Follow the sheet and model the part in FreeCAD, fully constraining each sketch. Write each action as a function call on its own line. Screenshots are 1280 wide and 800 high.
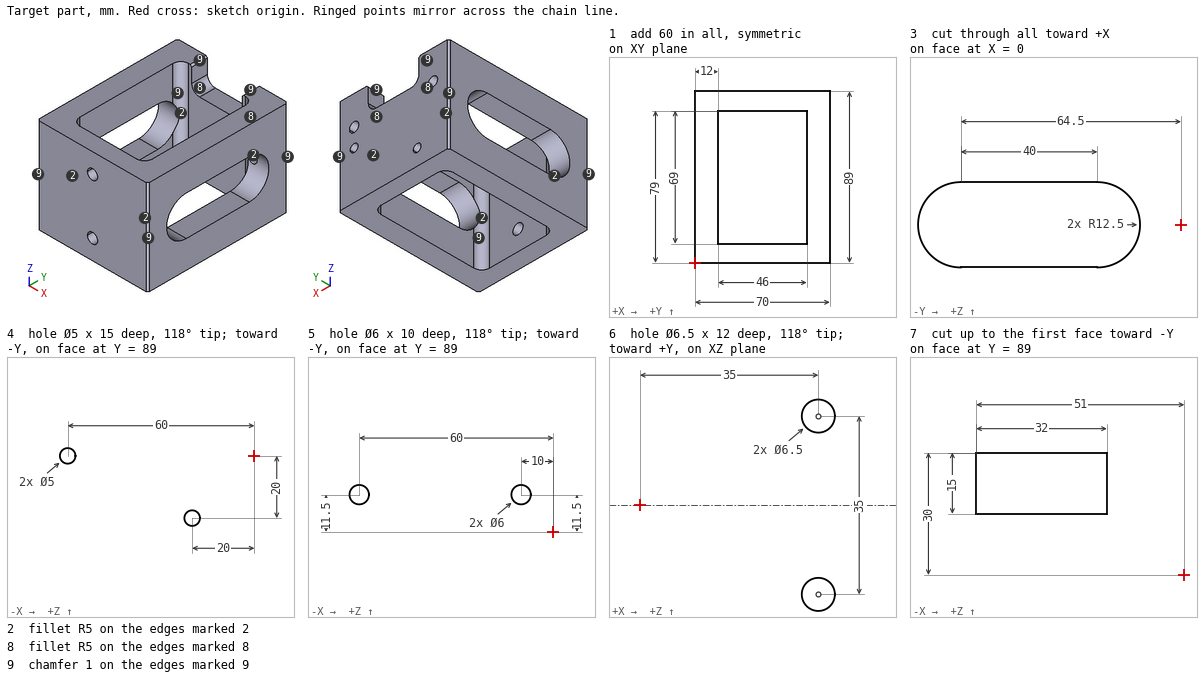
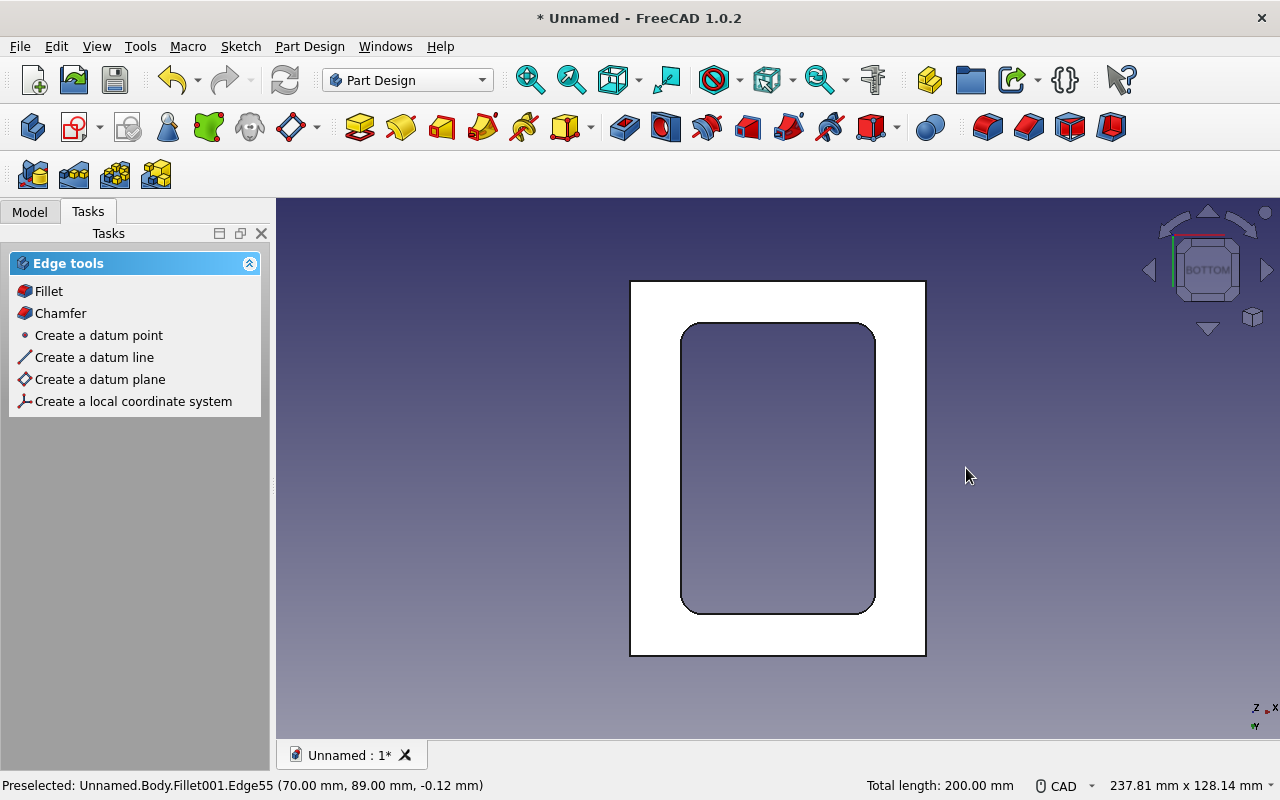
key(4)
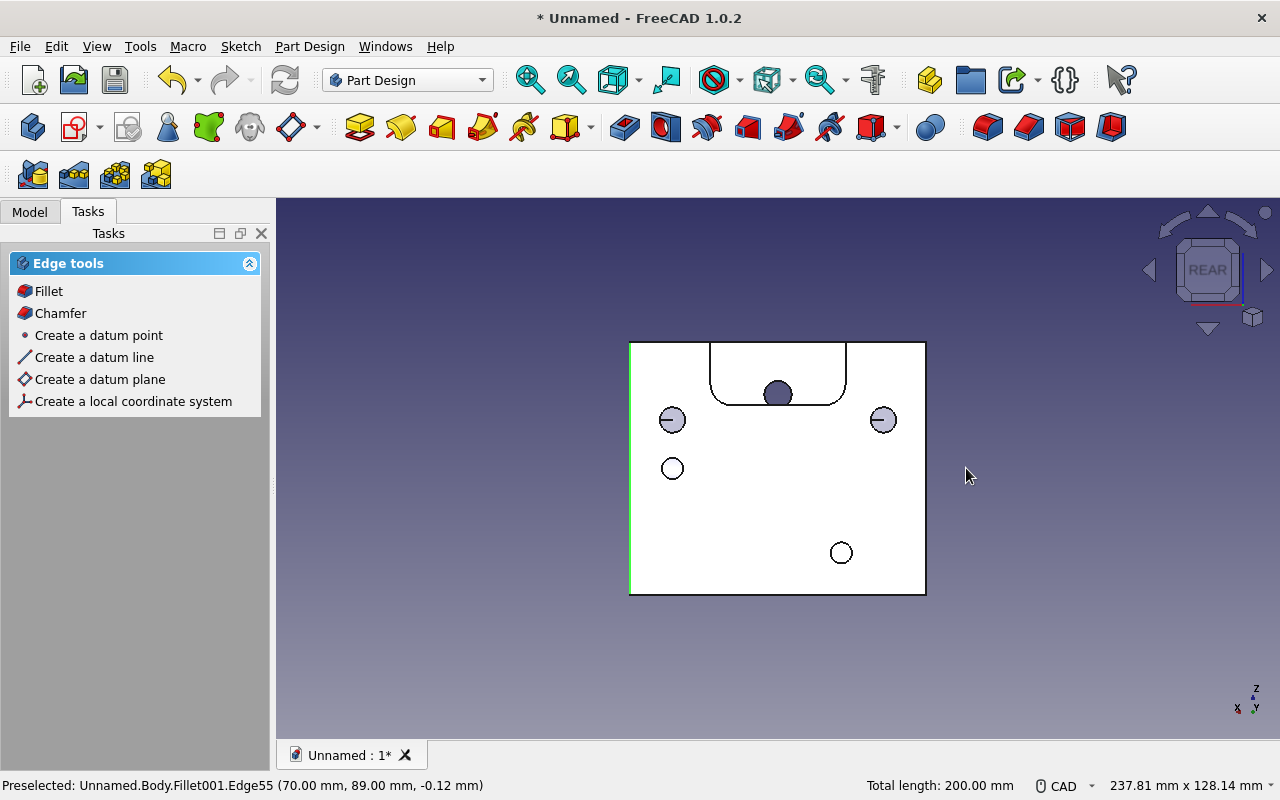
click(926, 468, ctrl)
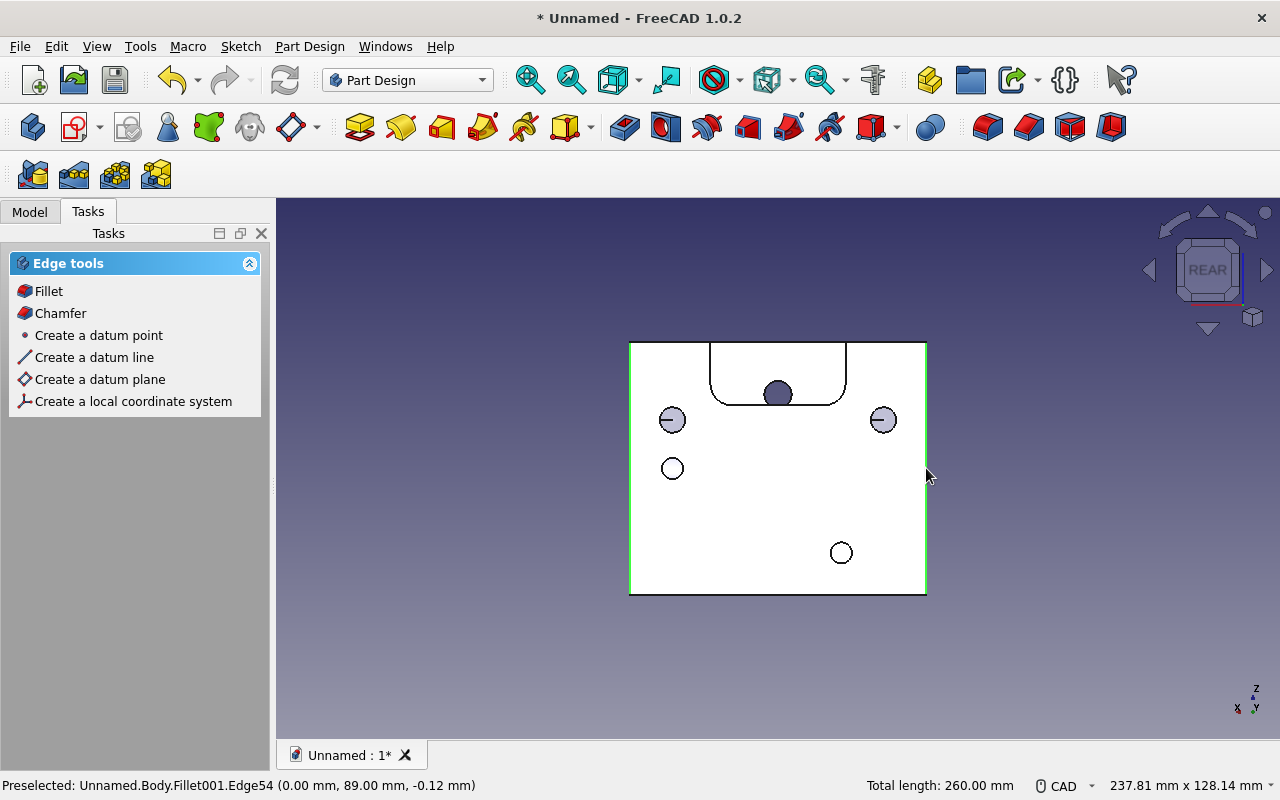
click(1029, 128)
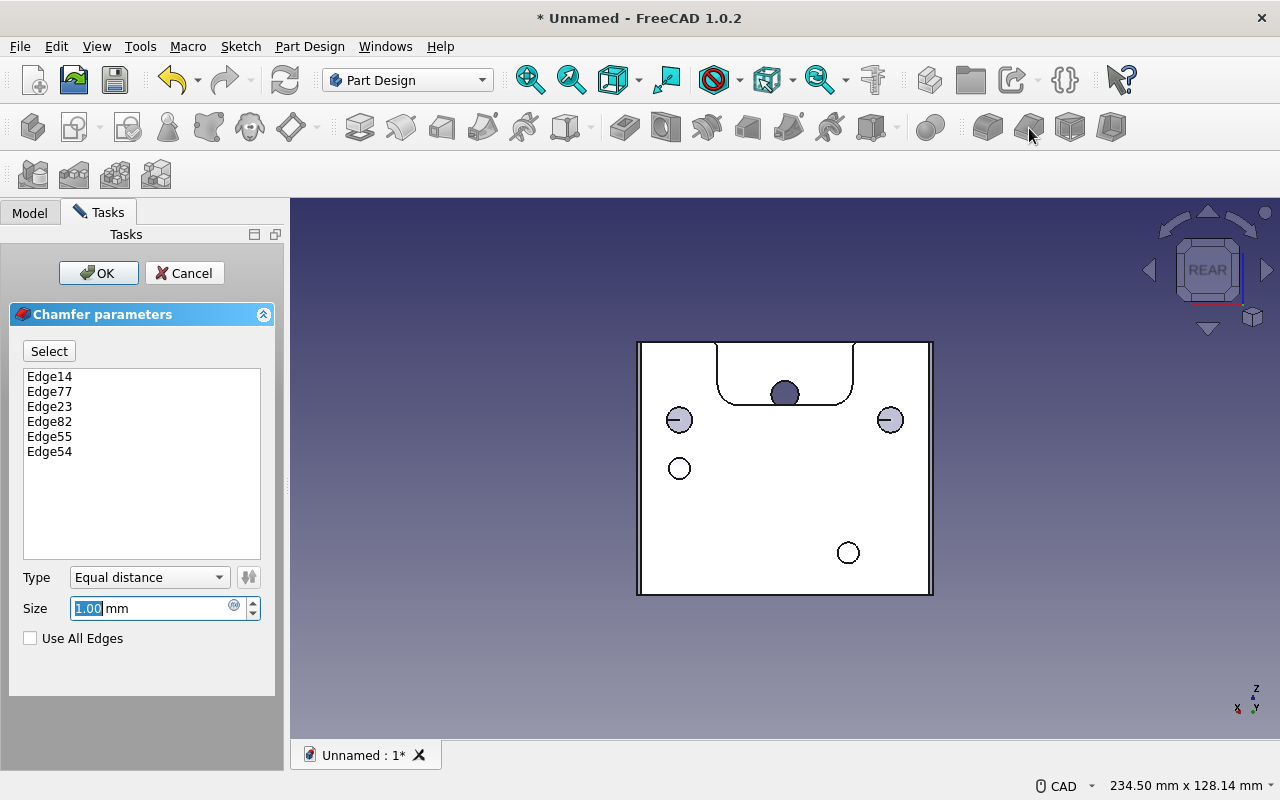
text(1)
key(Tab)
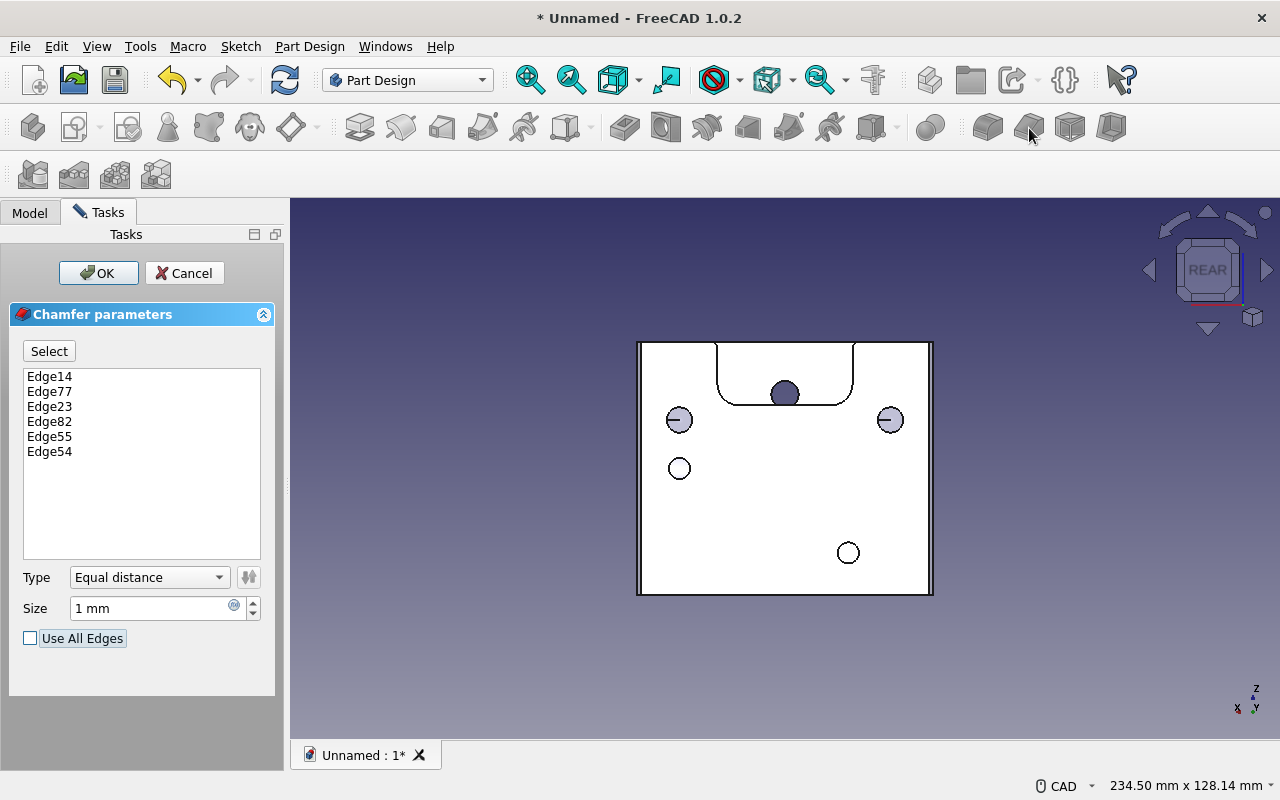
click(99, 273)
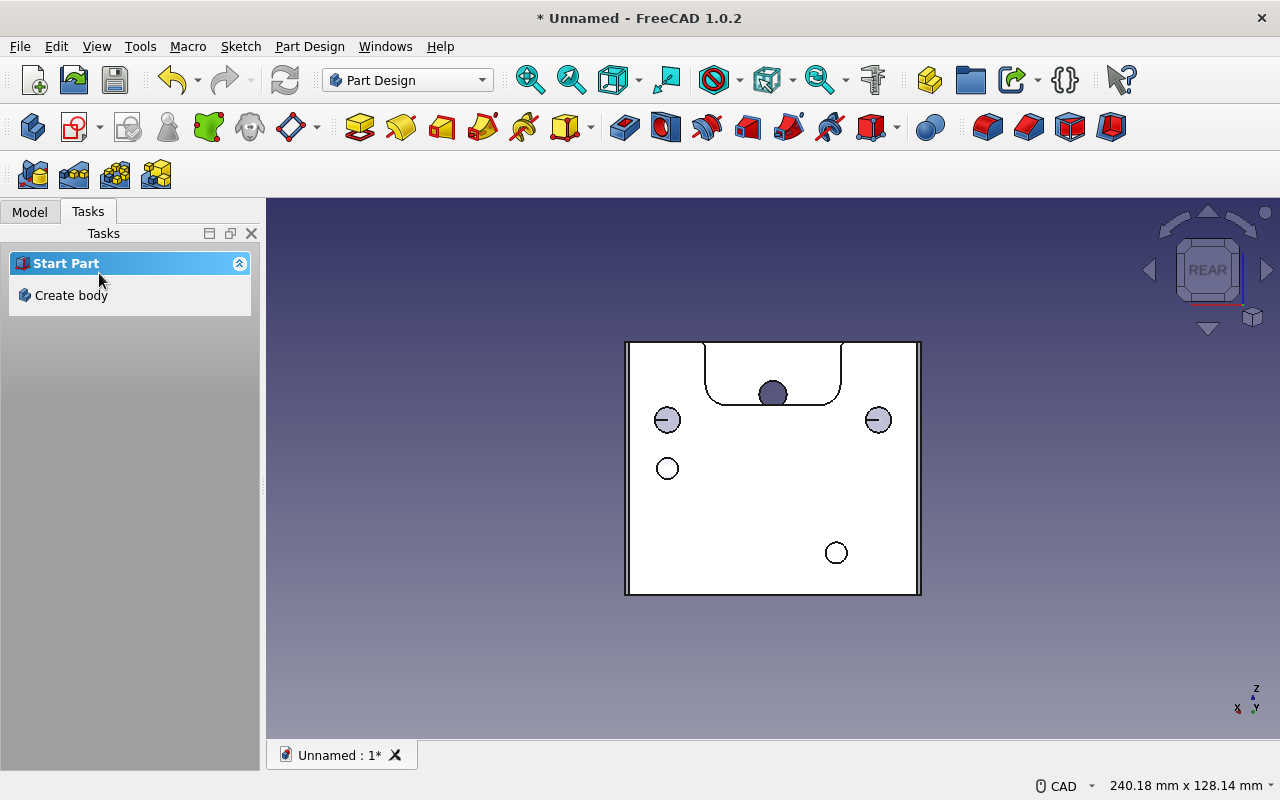
key(0)